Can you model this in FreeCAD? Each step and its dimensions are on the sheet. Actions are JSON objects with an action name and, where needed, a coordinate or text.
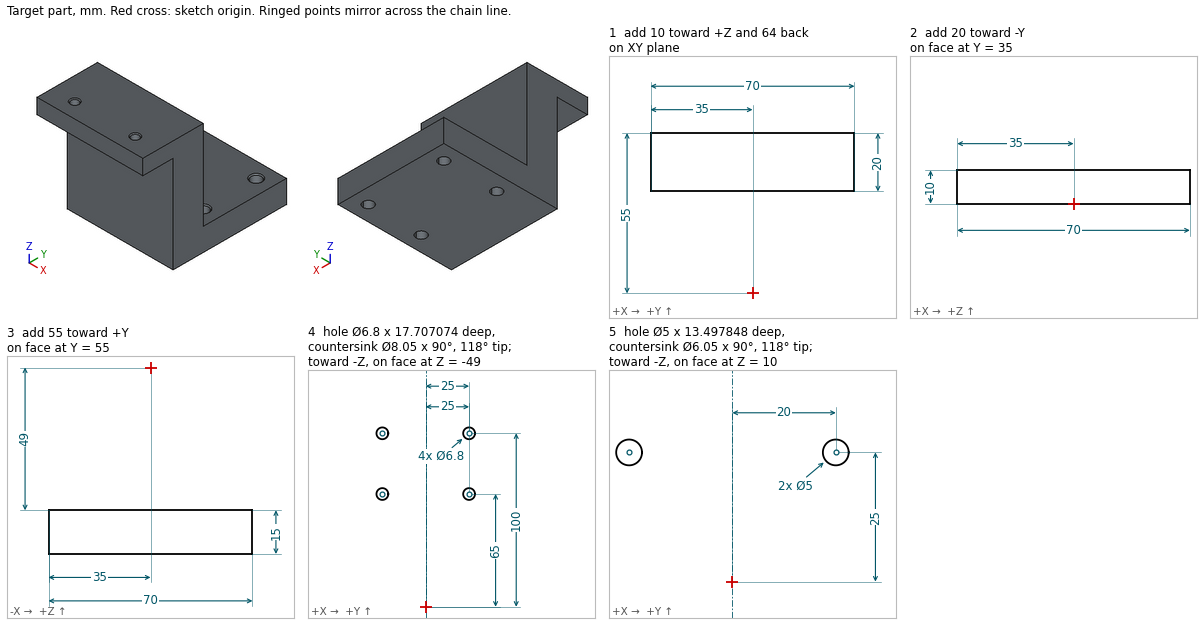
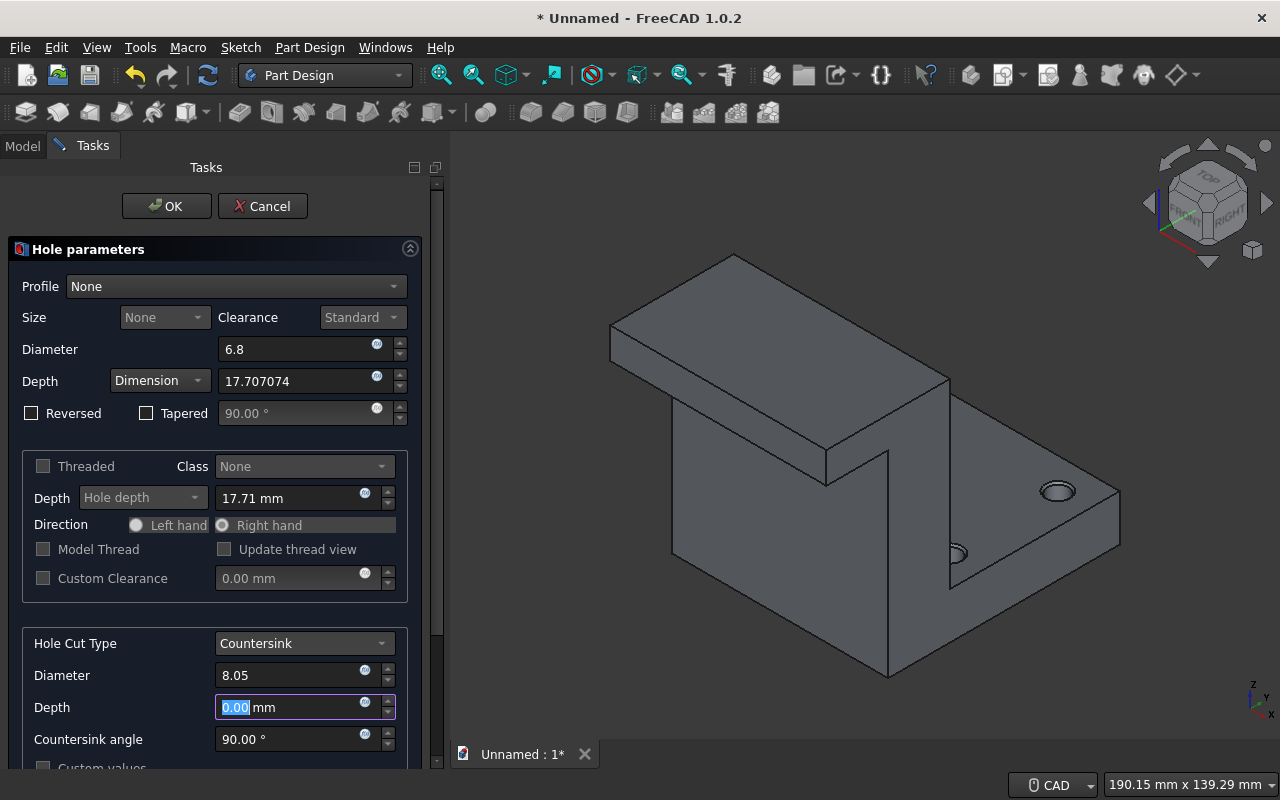
{"action": "left_click", "coordinate": [167, 206]}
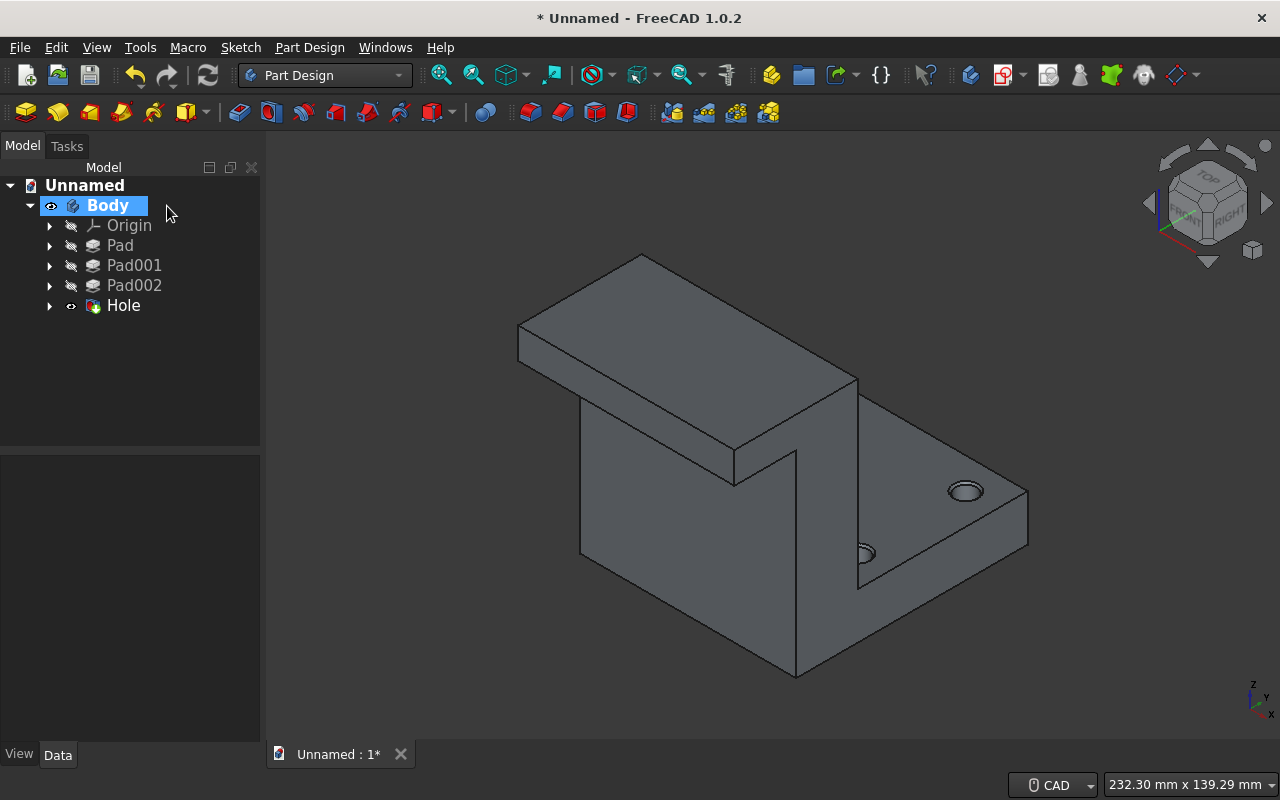
{"action": "left_click", "coordinate": [719, 369]}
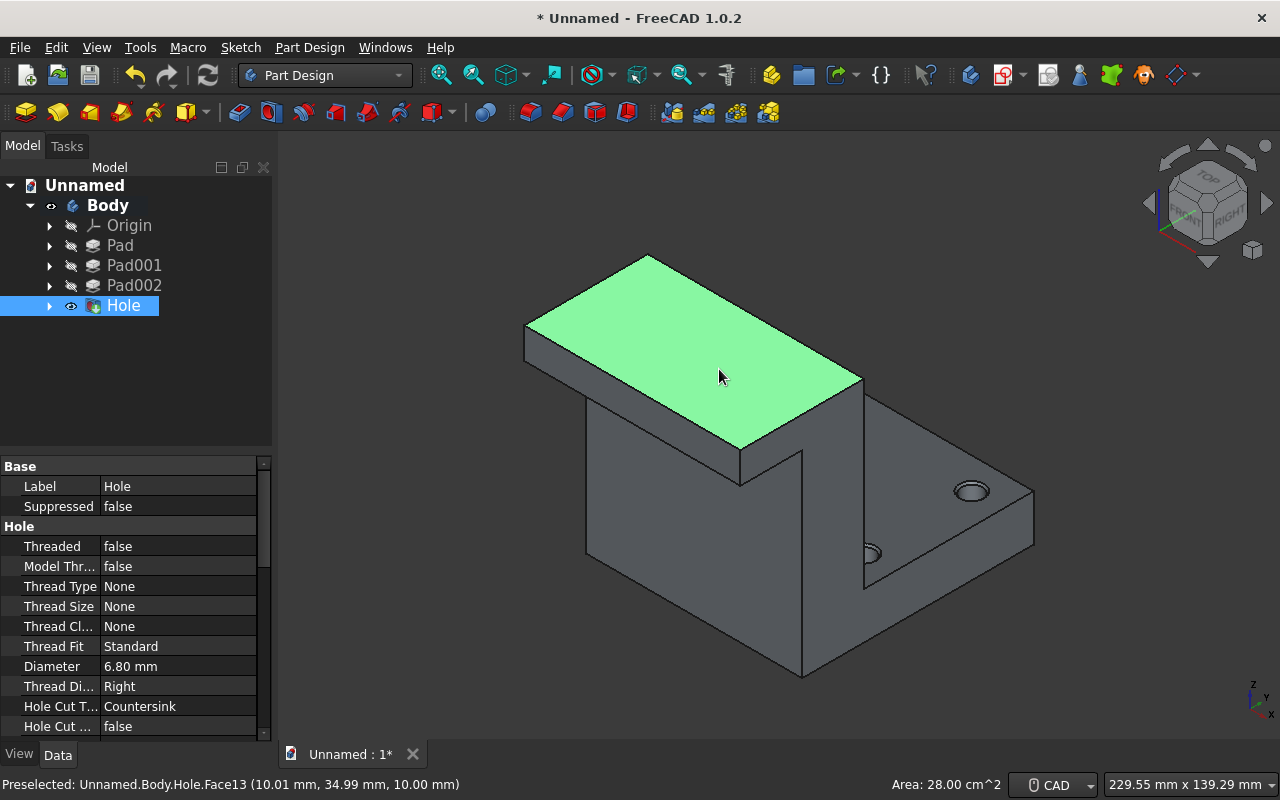
{"action": "left_click", "coordinate": [1004, 76]}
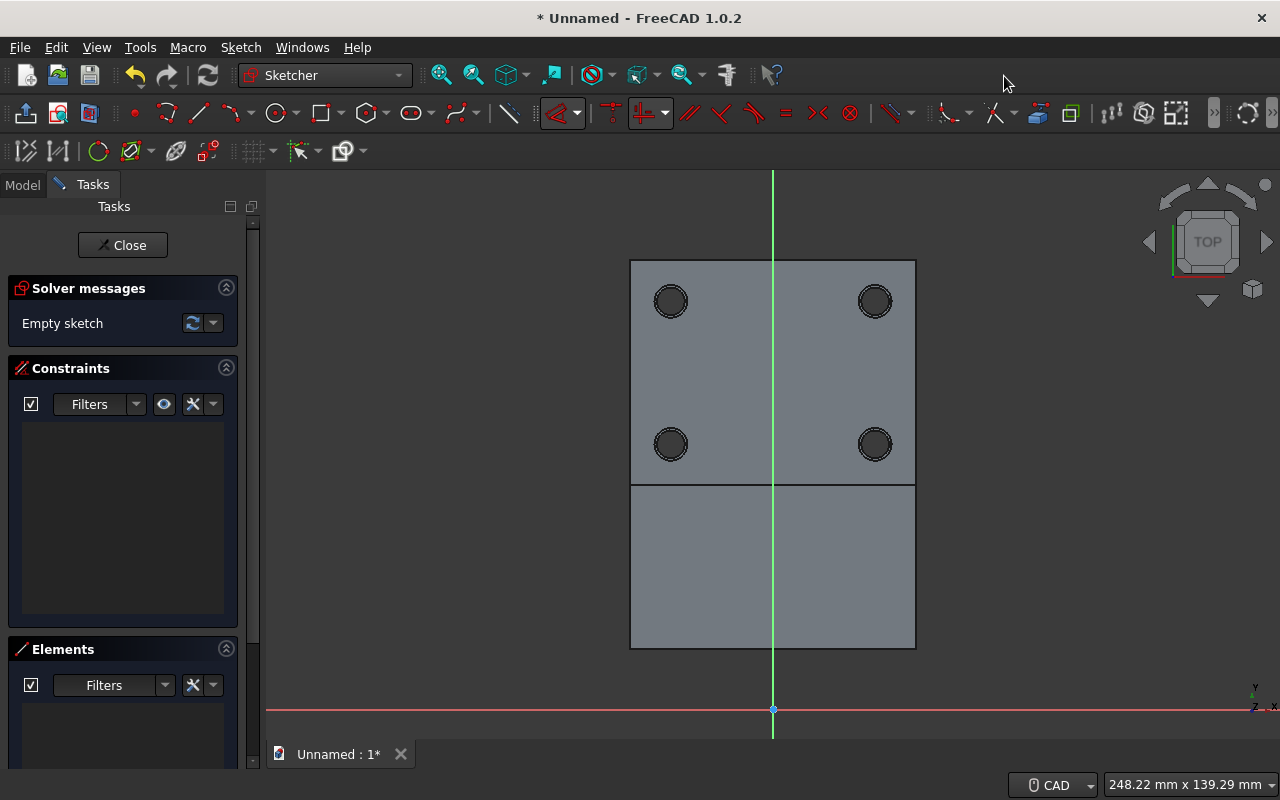
{"action": "scroll", "coordinate": [704, 454], "scroll_direction": "down", "scroll_amount": 5}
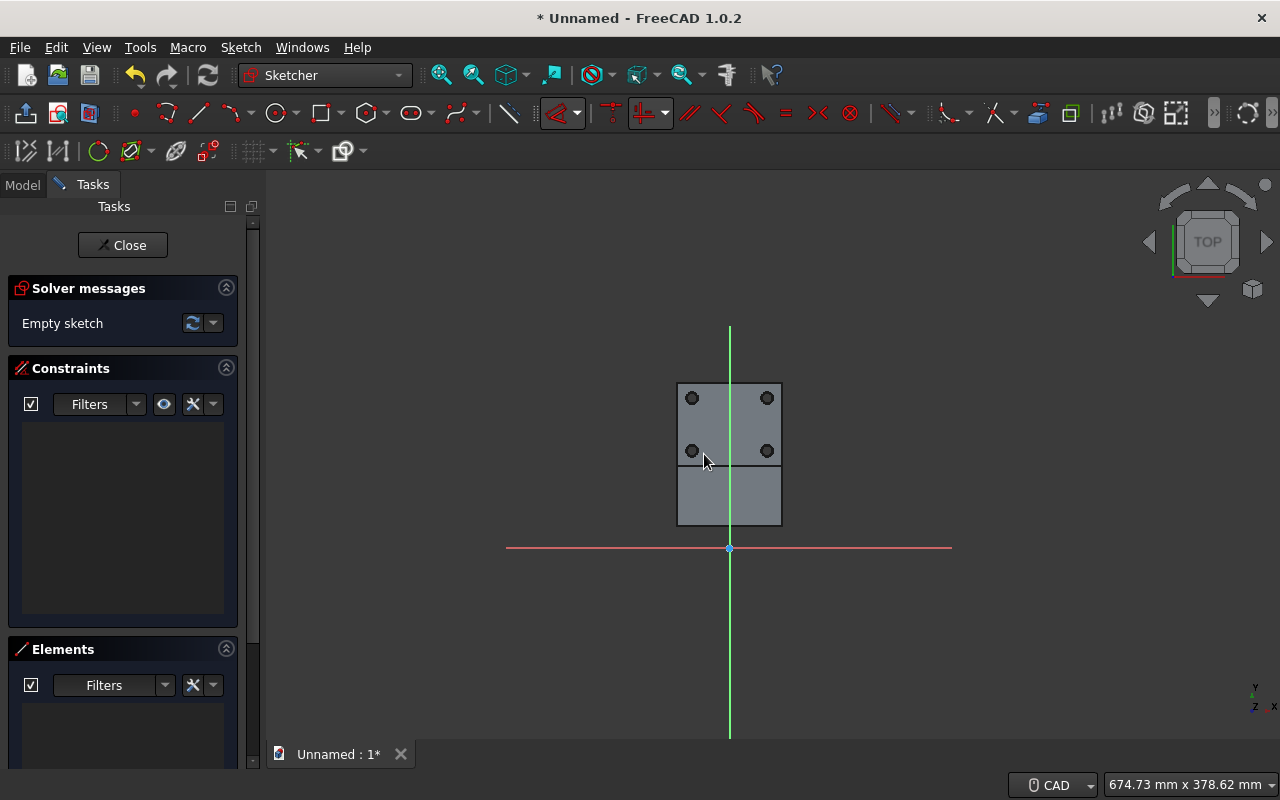
{"action": "scroll", "coordinate": [733, 537], "scroll_direction": "up", "scroll_amount": 11}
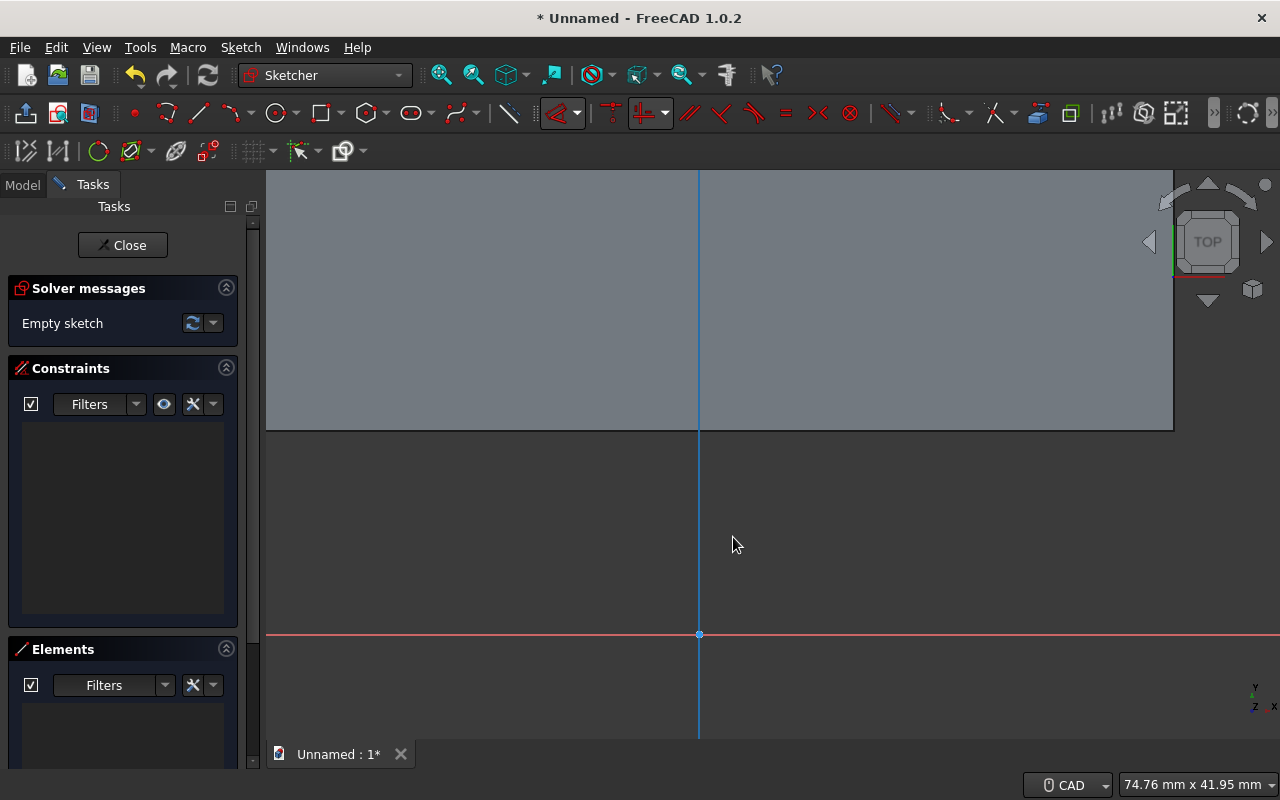
{"action": "left_click", "coordinate": [276, 114]}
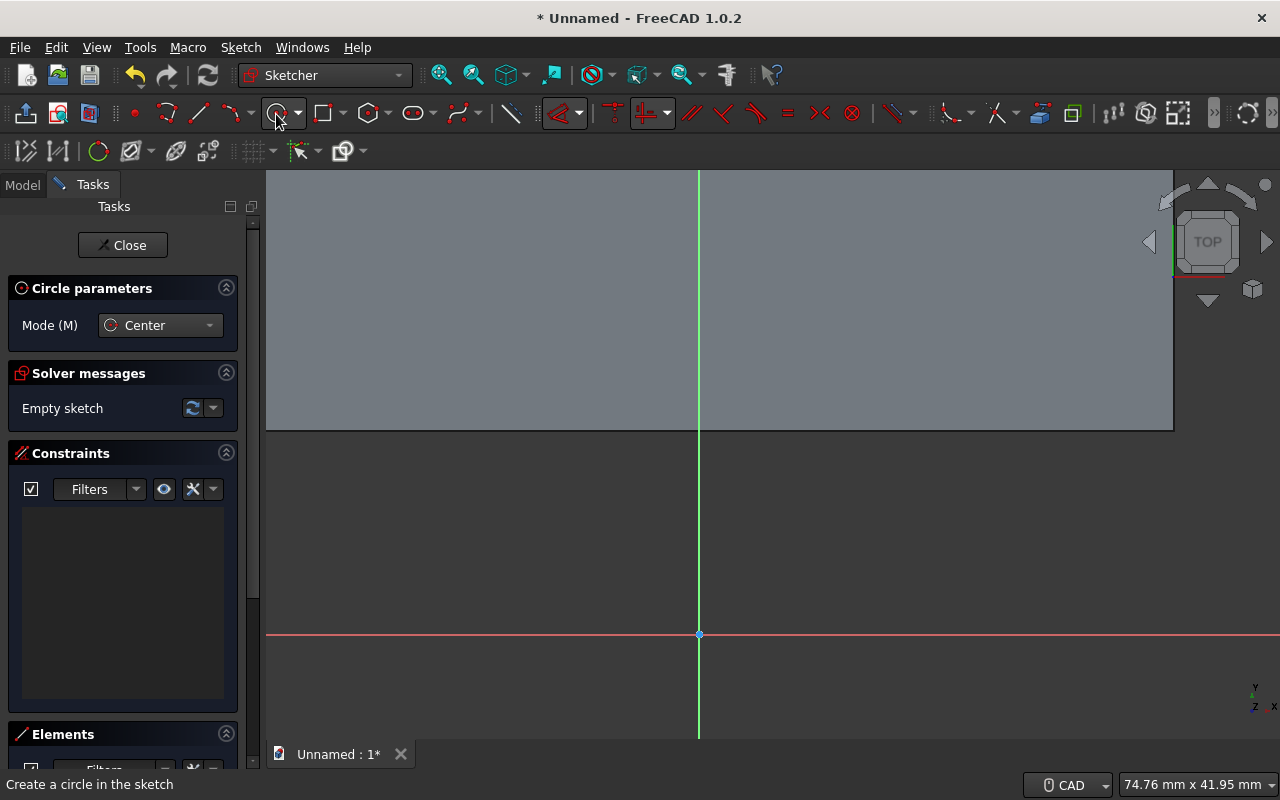
{"action": "left_click", "coordinate": [970, 296]}
{"action": "mouse_move", "coordinate": [994, 272]}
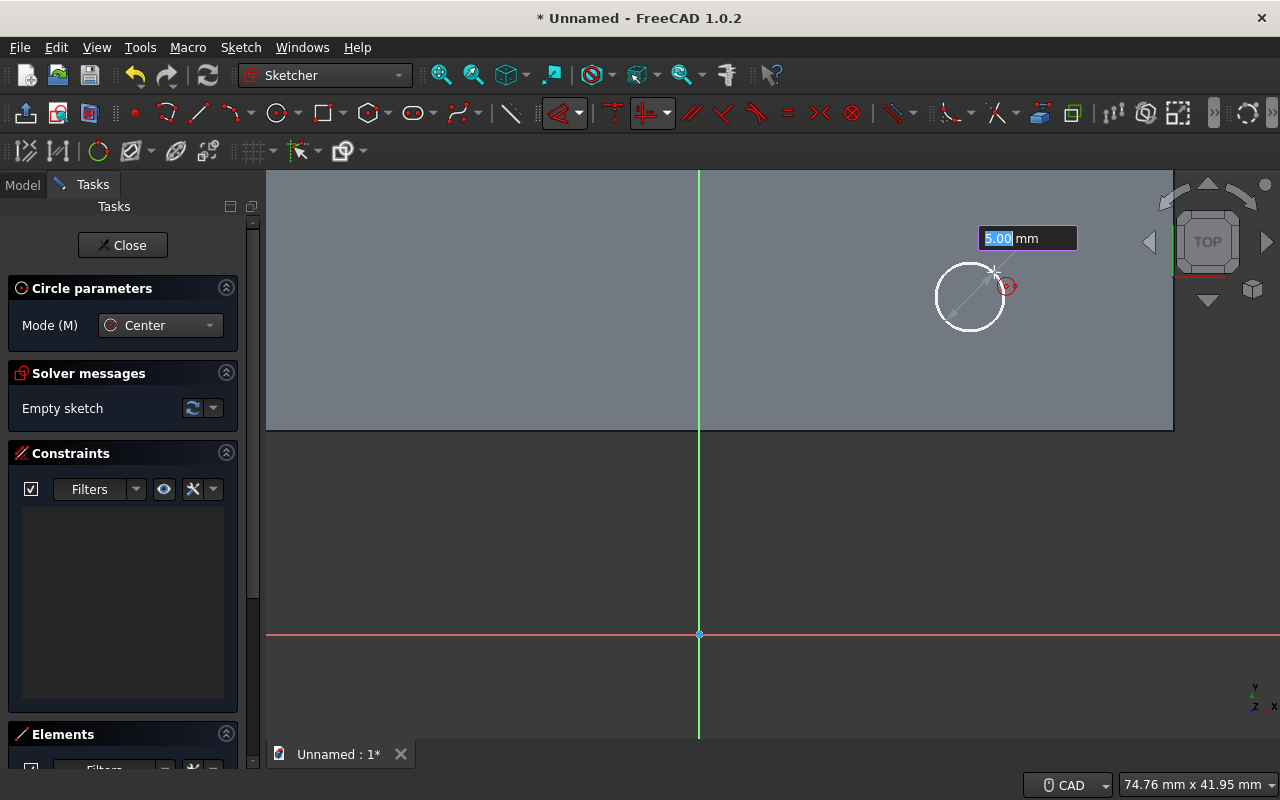
{"action": "type", "text": "5"}
{"action": "key", "text": "Return"}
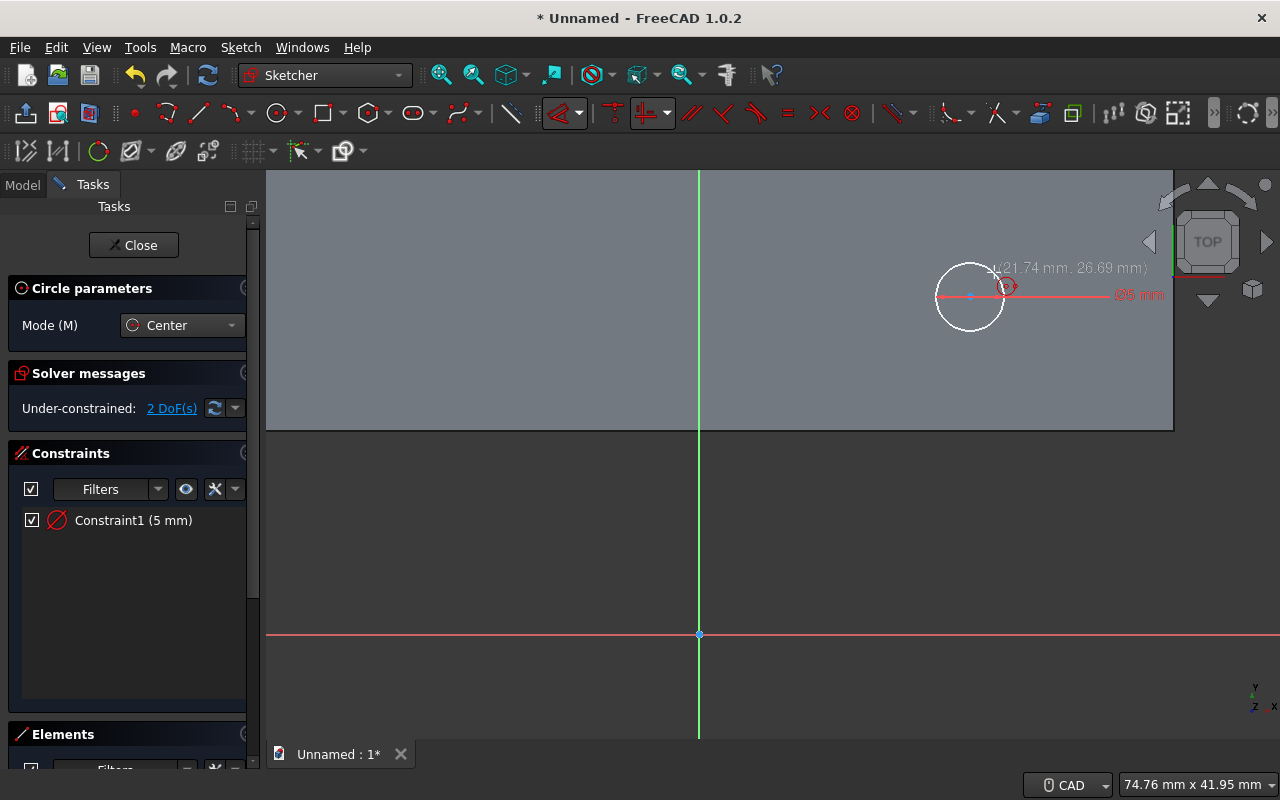
{"action": "left_click", "coordinate": [428, 296]}
{"action": "mouse_move", "coordinate": [452, 272]}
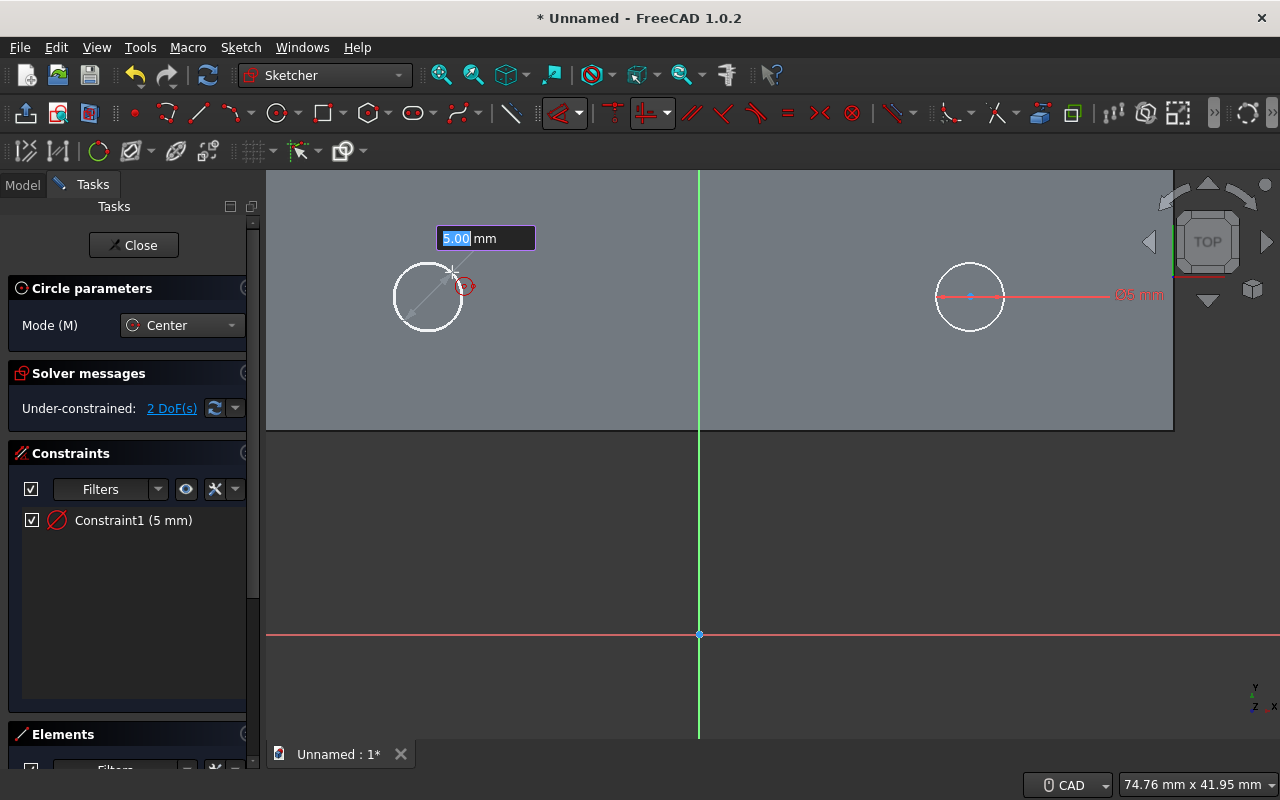
{"action": "type", "text": "5"}
{"action": "key", "text": "Return"}
{"action": "key", "text": "Escape"}